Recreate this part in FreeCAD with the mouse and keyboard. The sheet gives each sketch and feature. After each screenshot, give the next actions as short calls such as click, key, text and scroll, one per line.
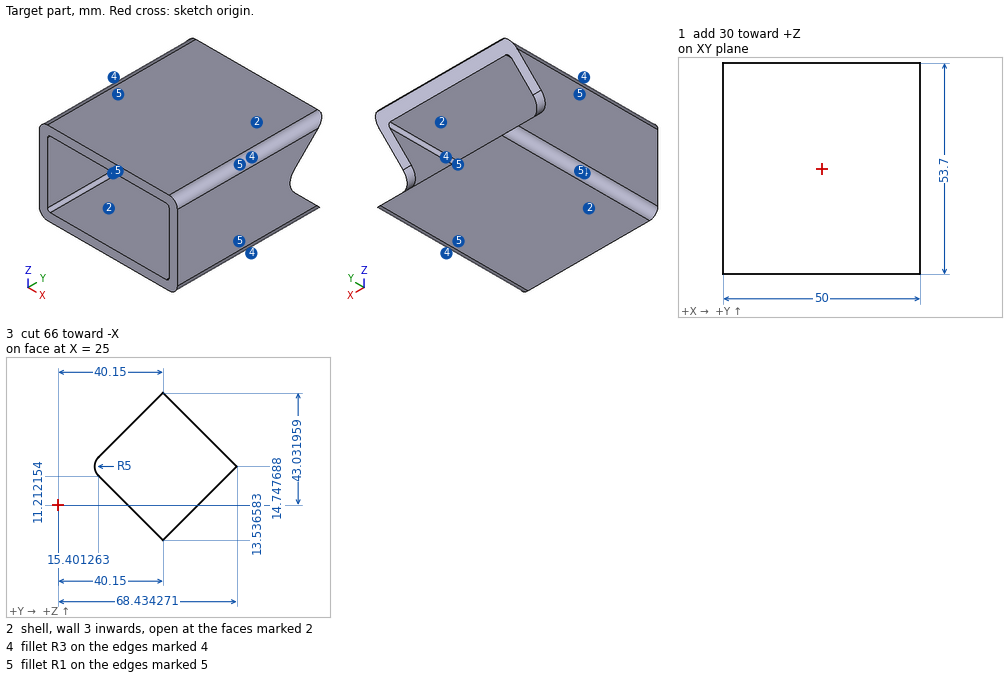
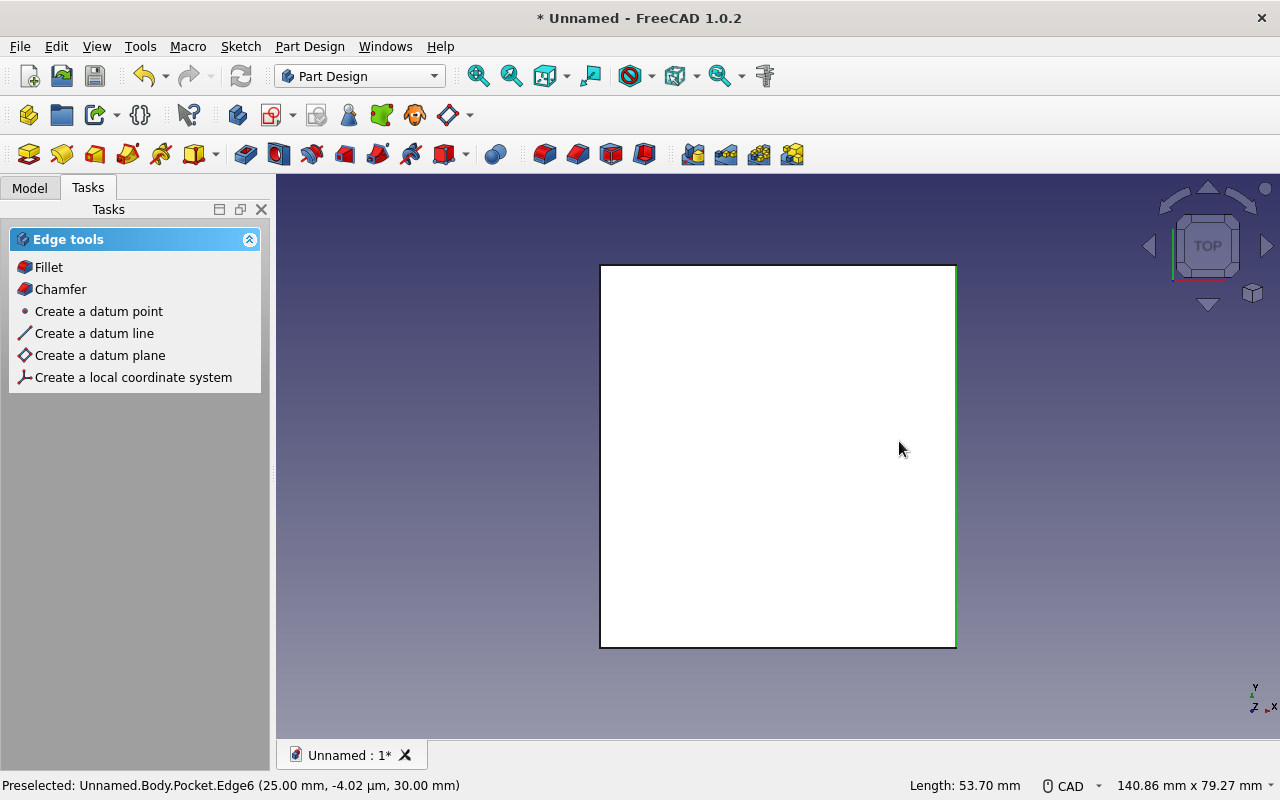
click(600, 455, ctrl)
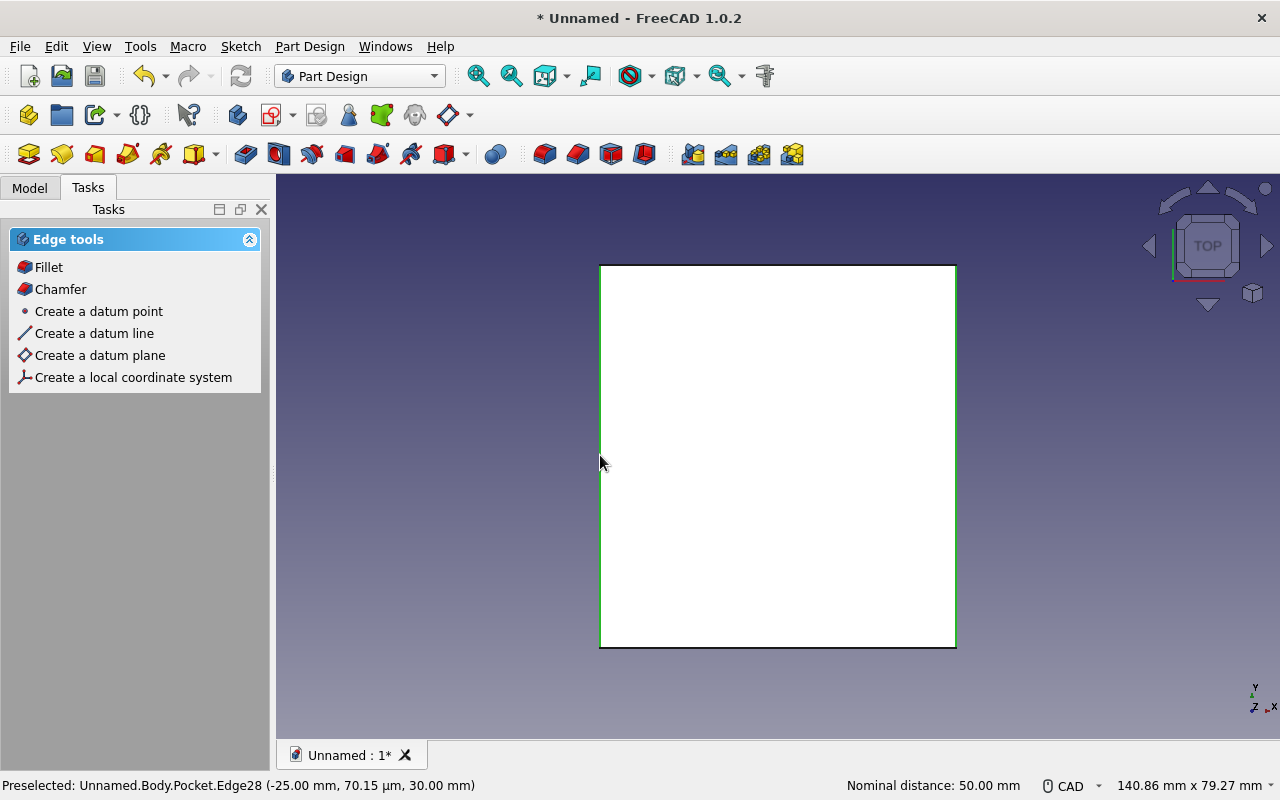
key(0)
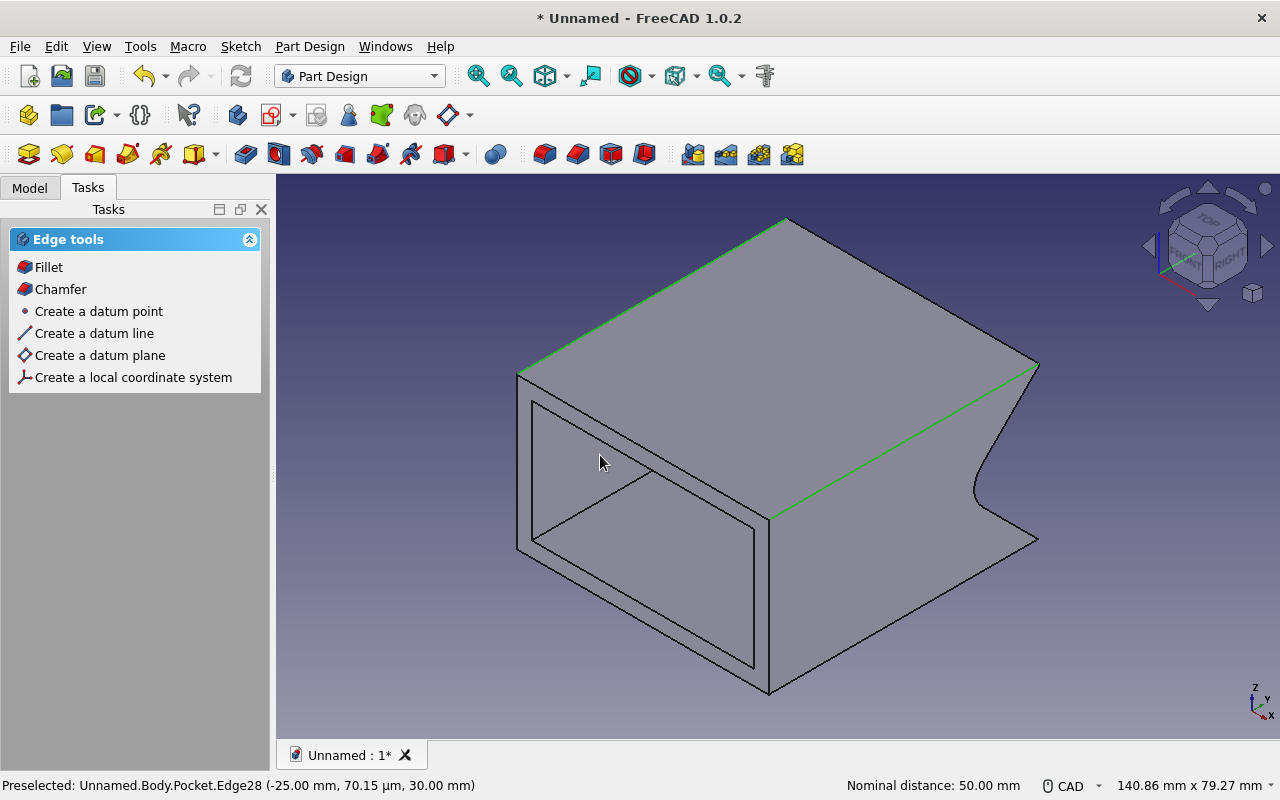
key(1)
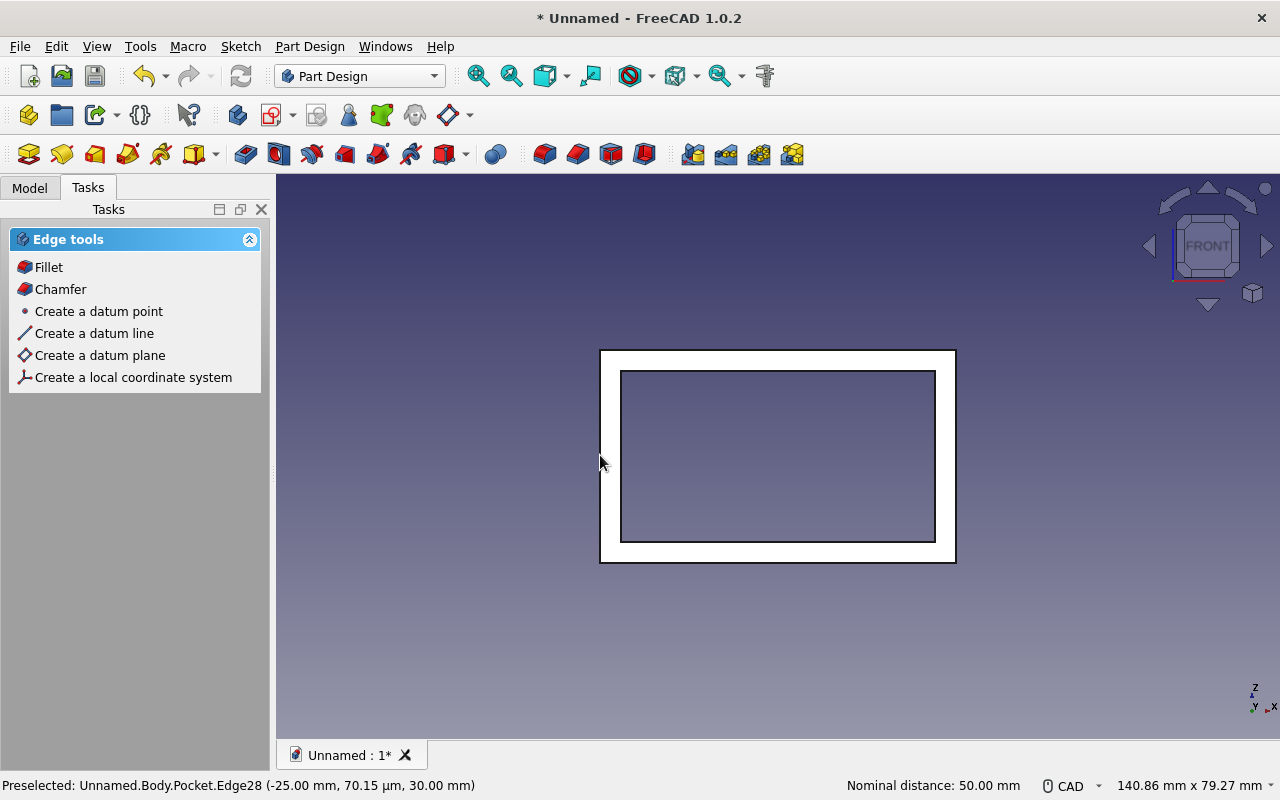
key(v)
key(f)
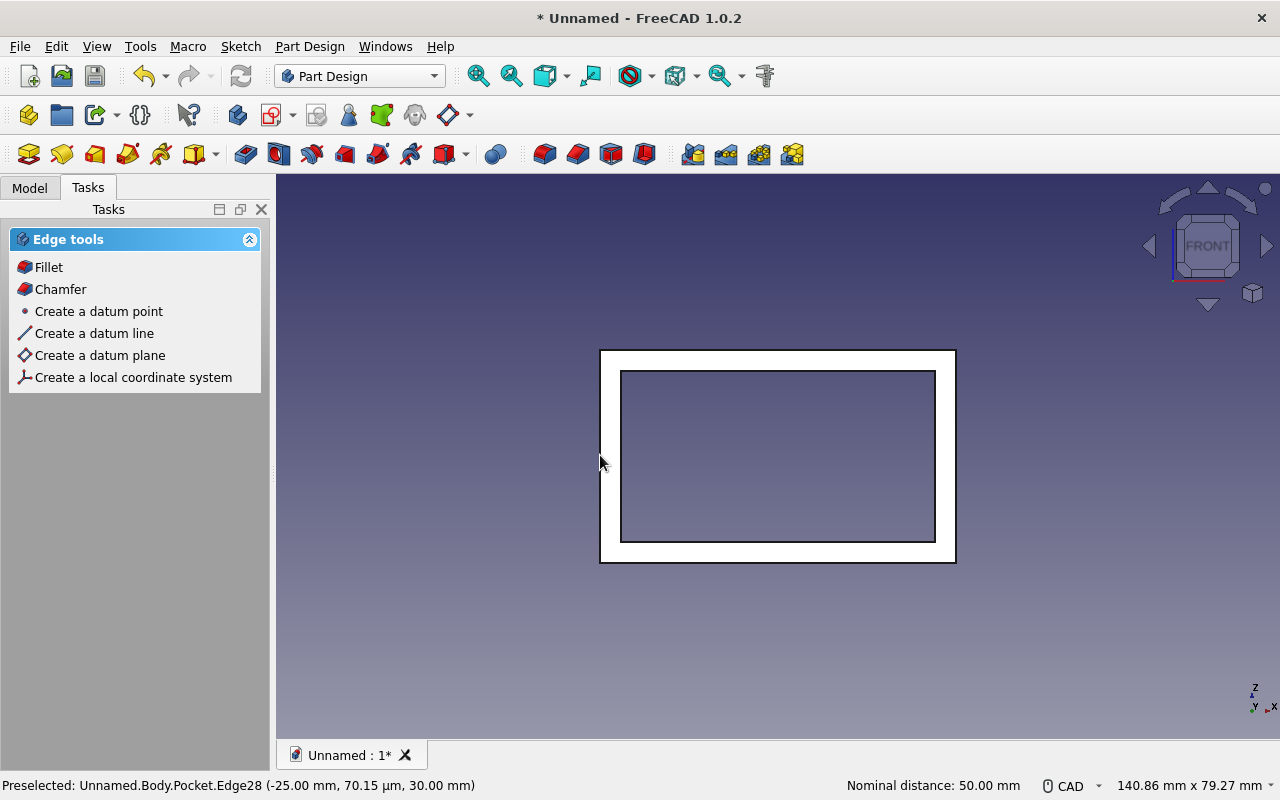
key(3)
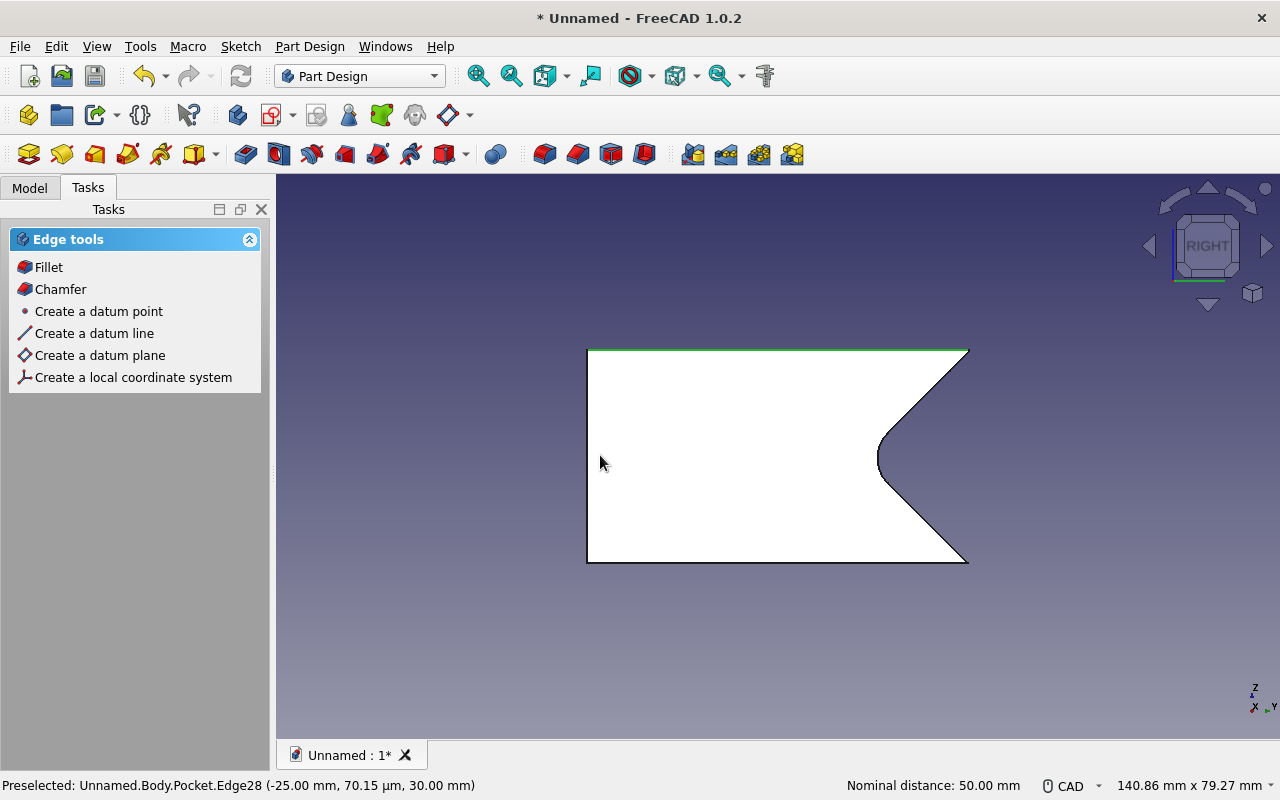
click(479, 76)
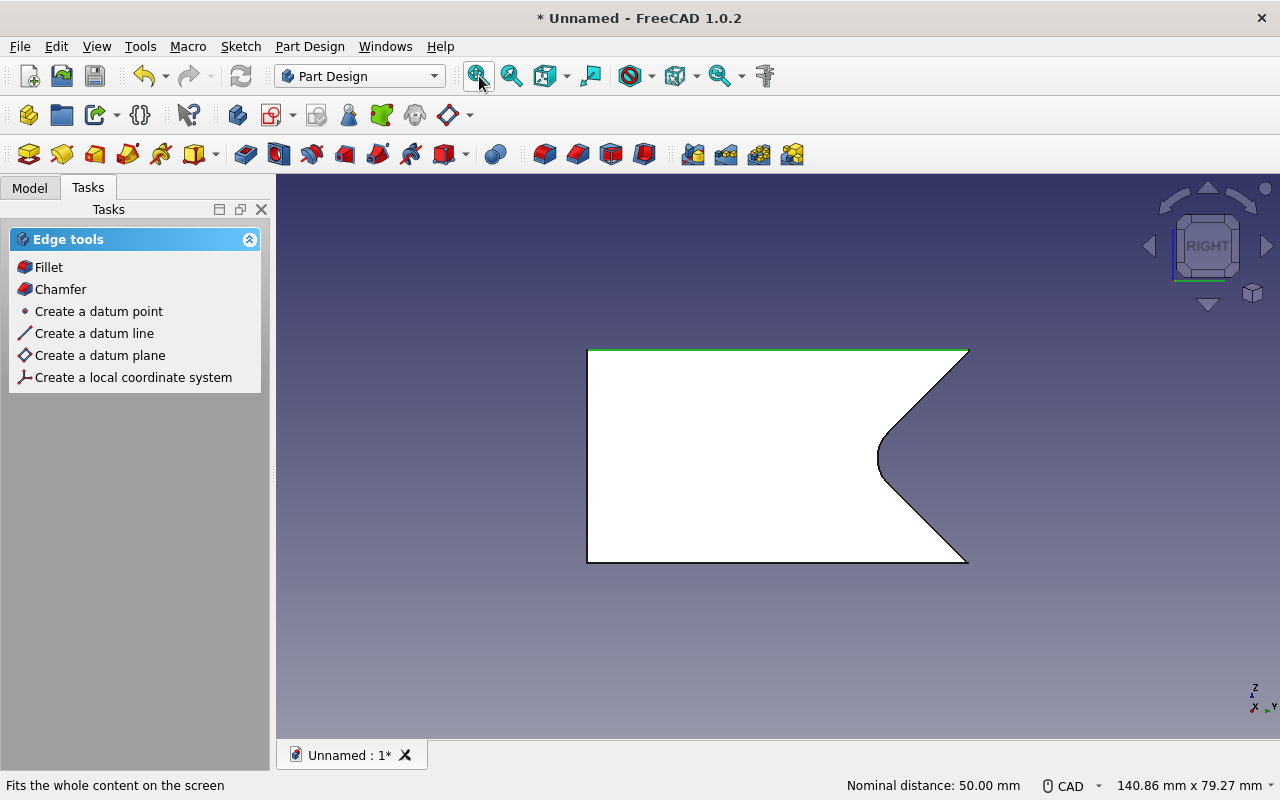
click(777, 562, ctrl)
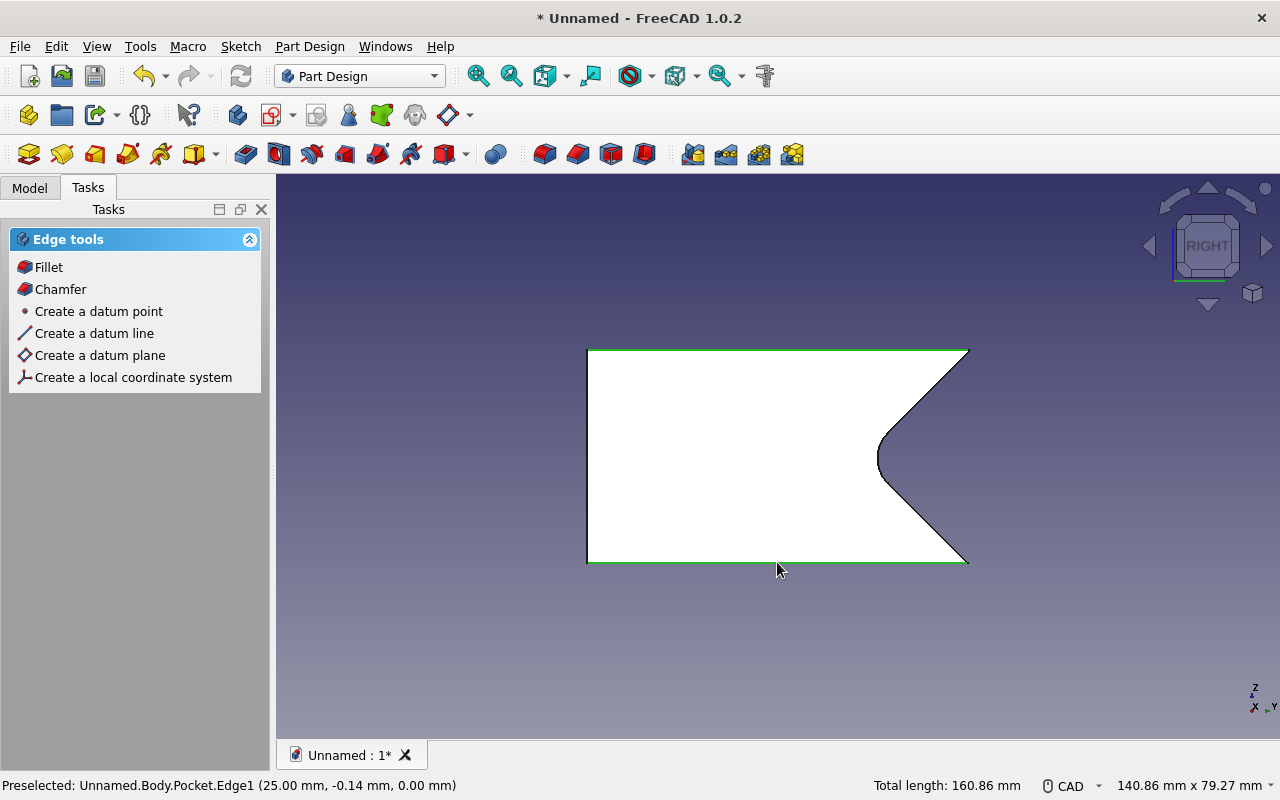
key(5)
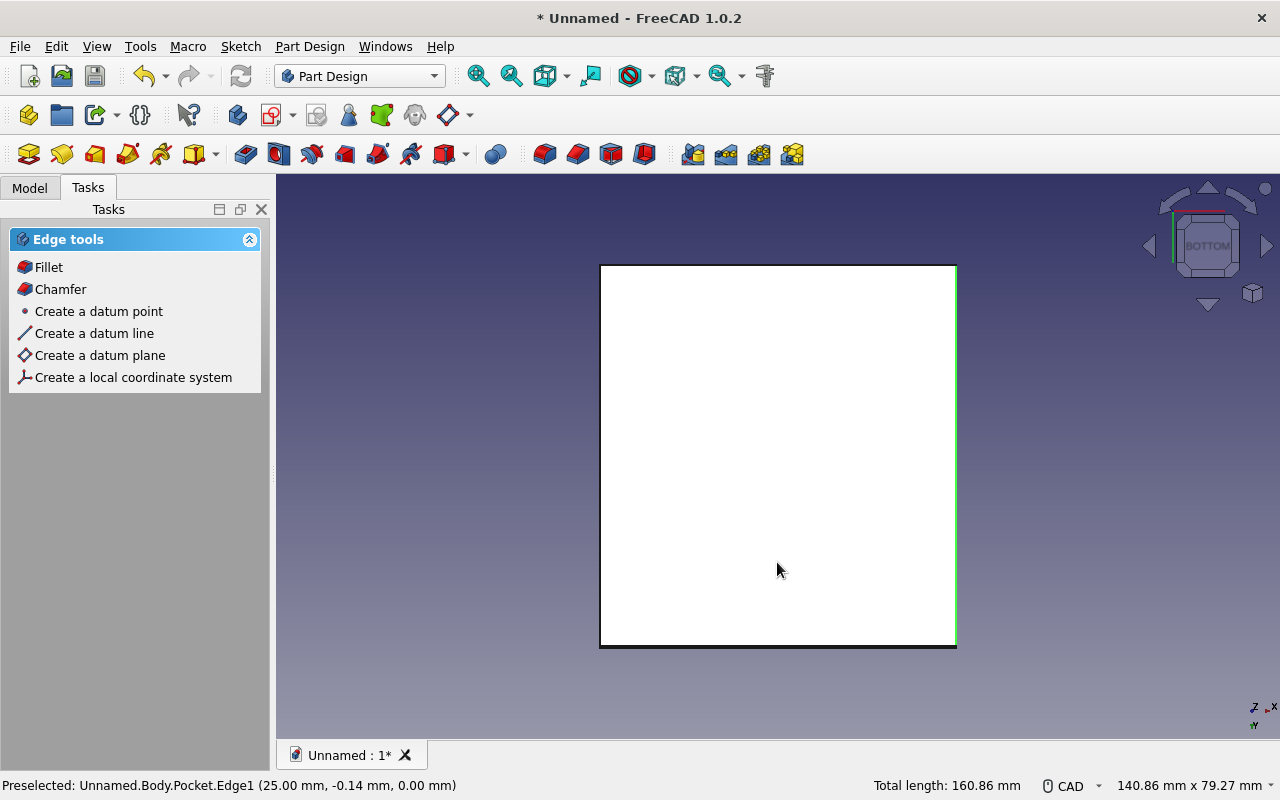
click(600, 455, ctrl)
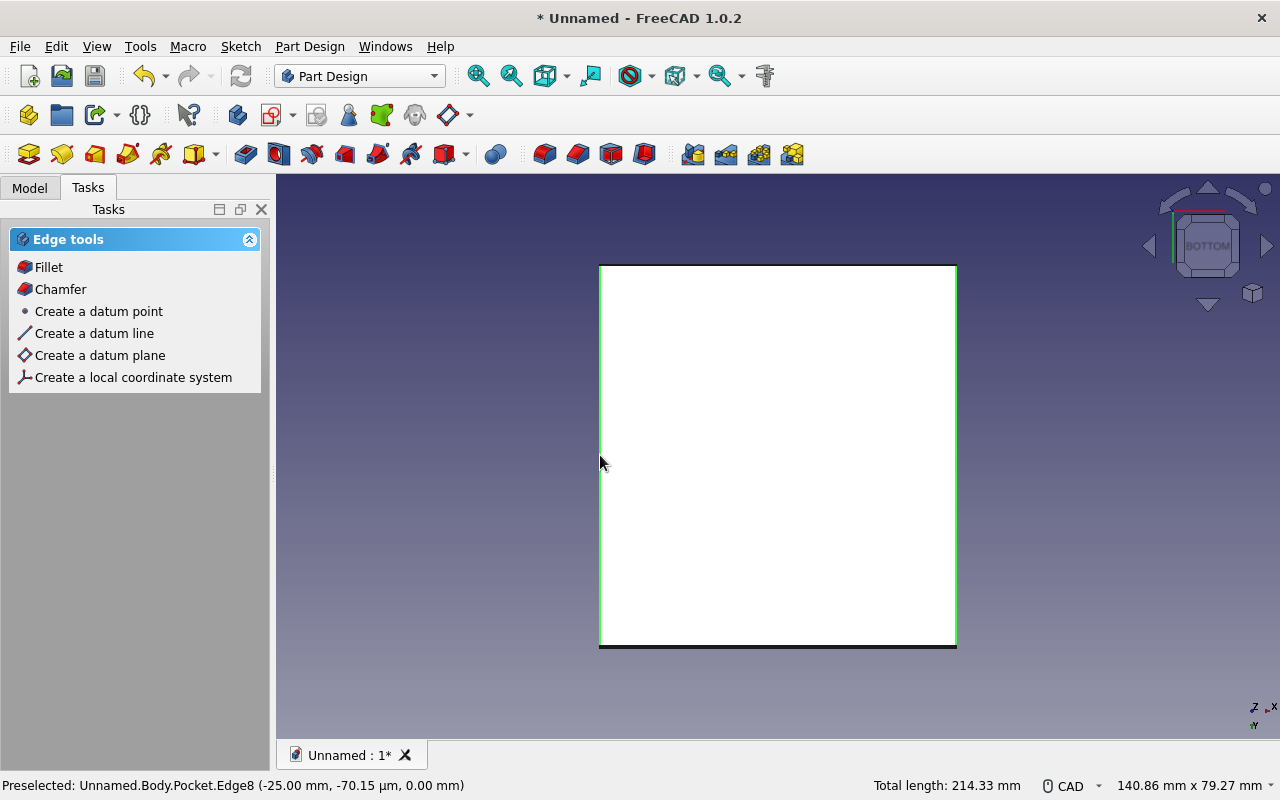
click(545, 154)